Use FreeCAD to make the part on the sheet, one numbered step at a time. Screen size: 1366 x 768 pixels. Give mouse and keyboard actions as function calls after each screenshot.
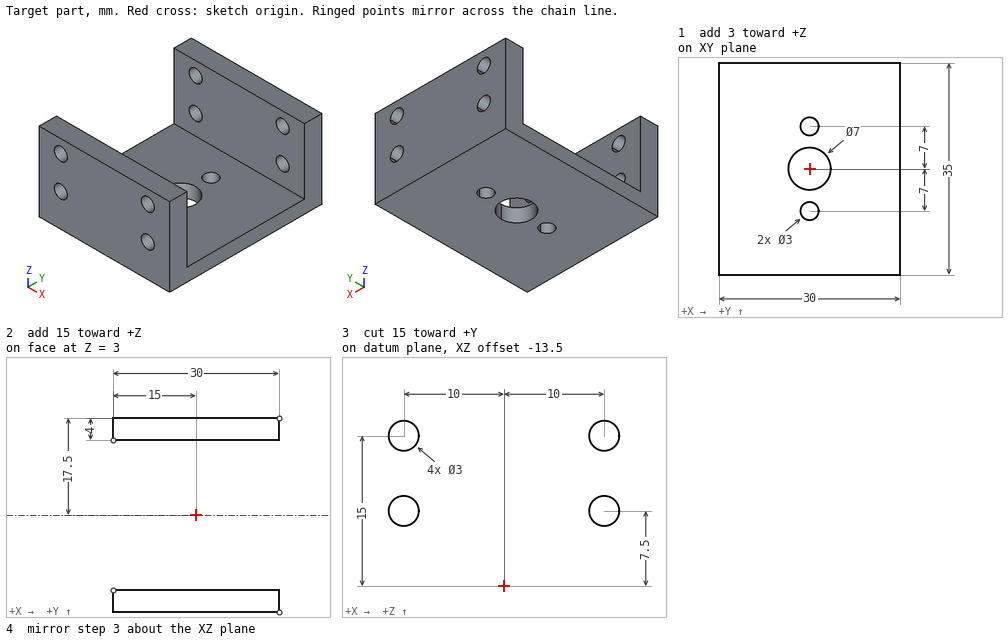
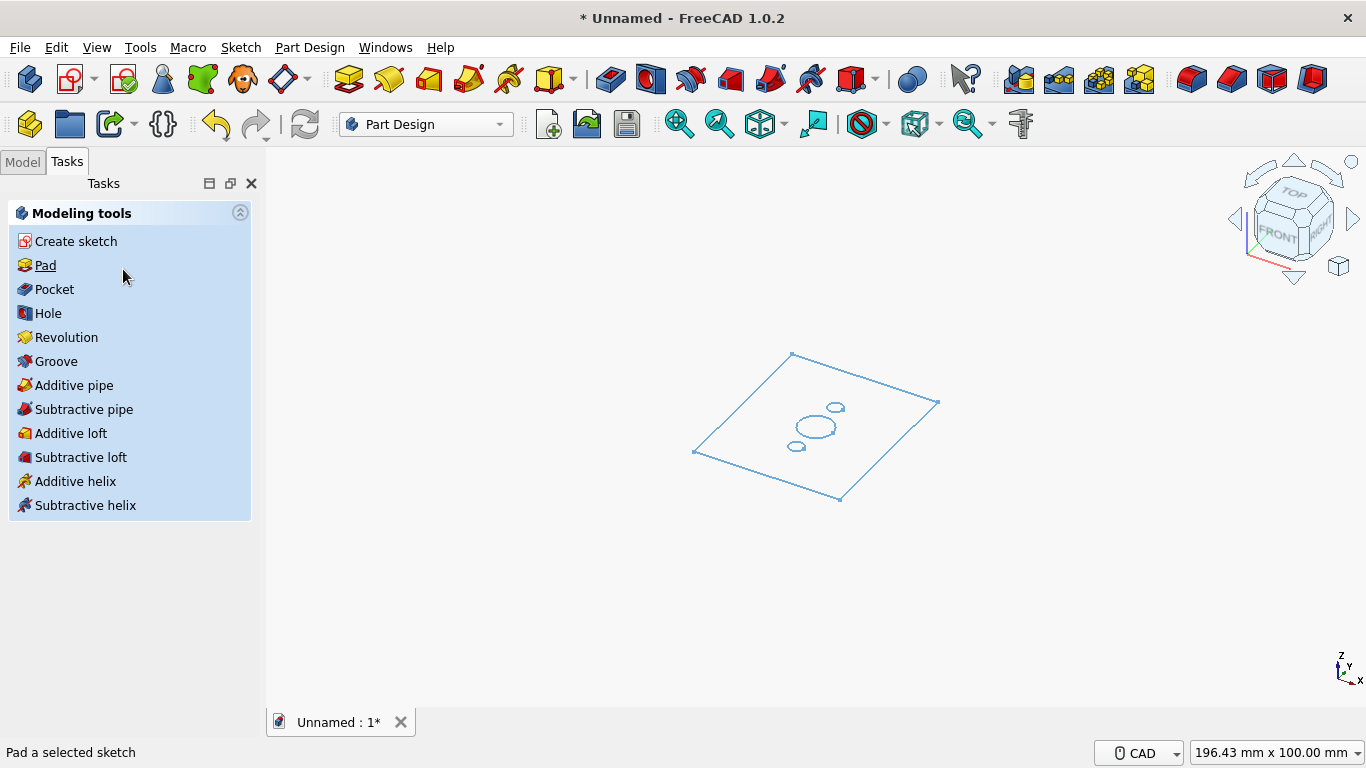
click(350, 80)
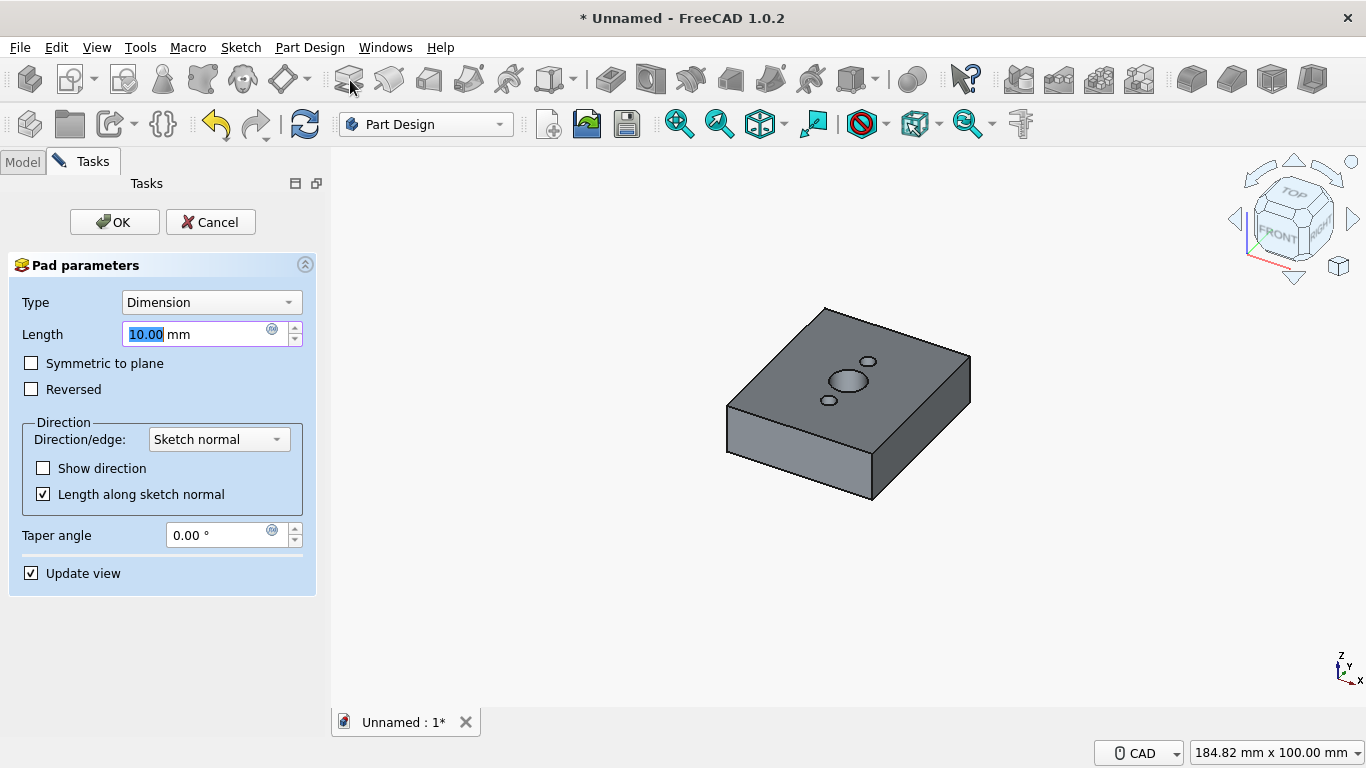
text(3)
key(Tab)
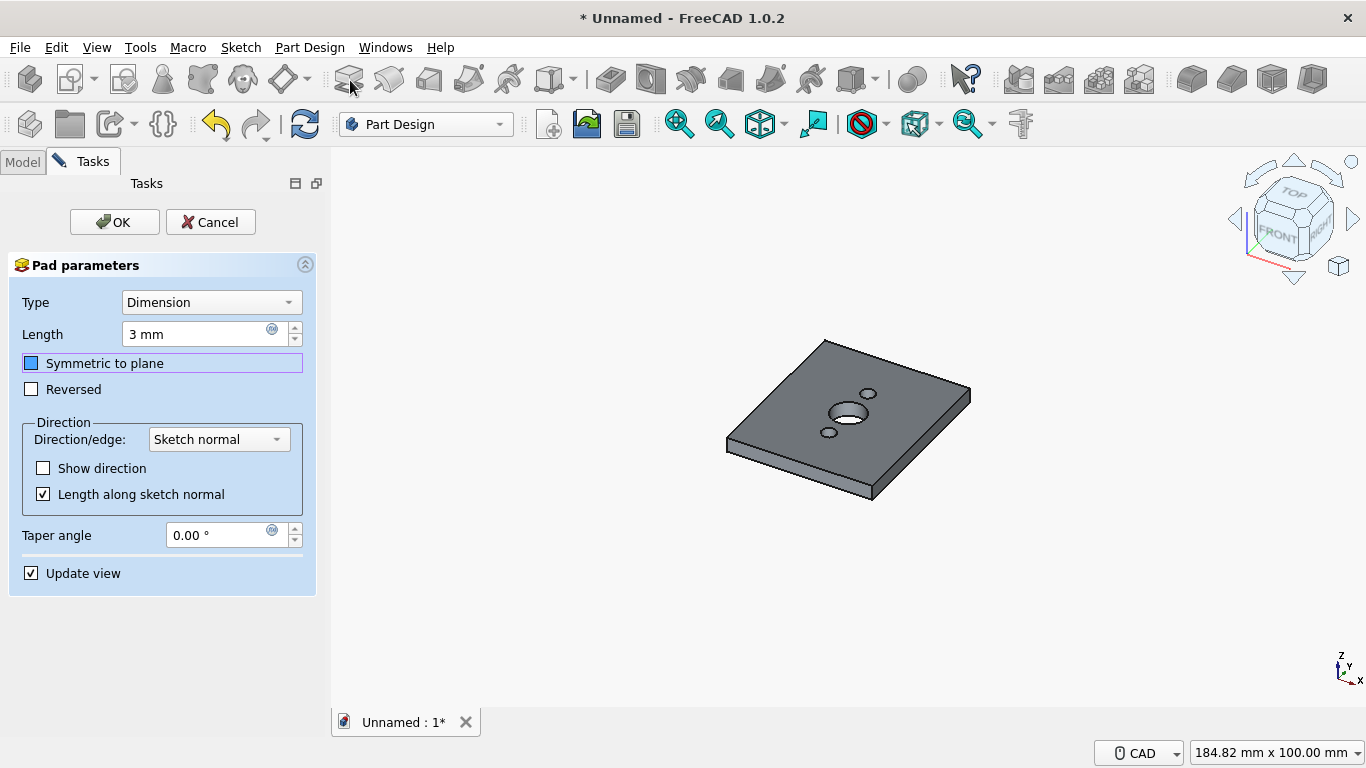
click(115, 222)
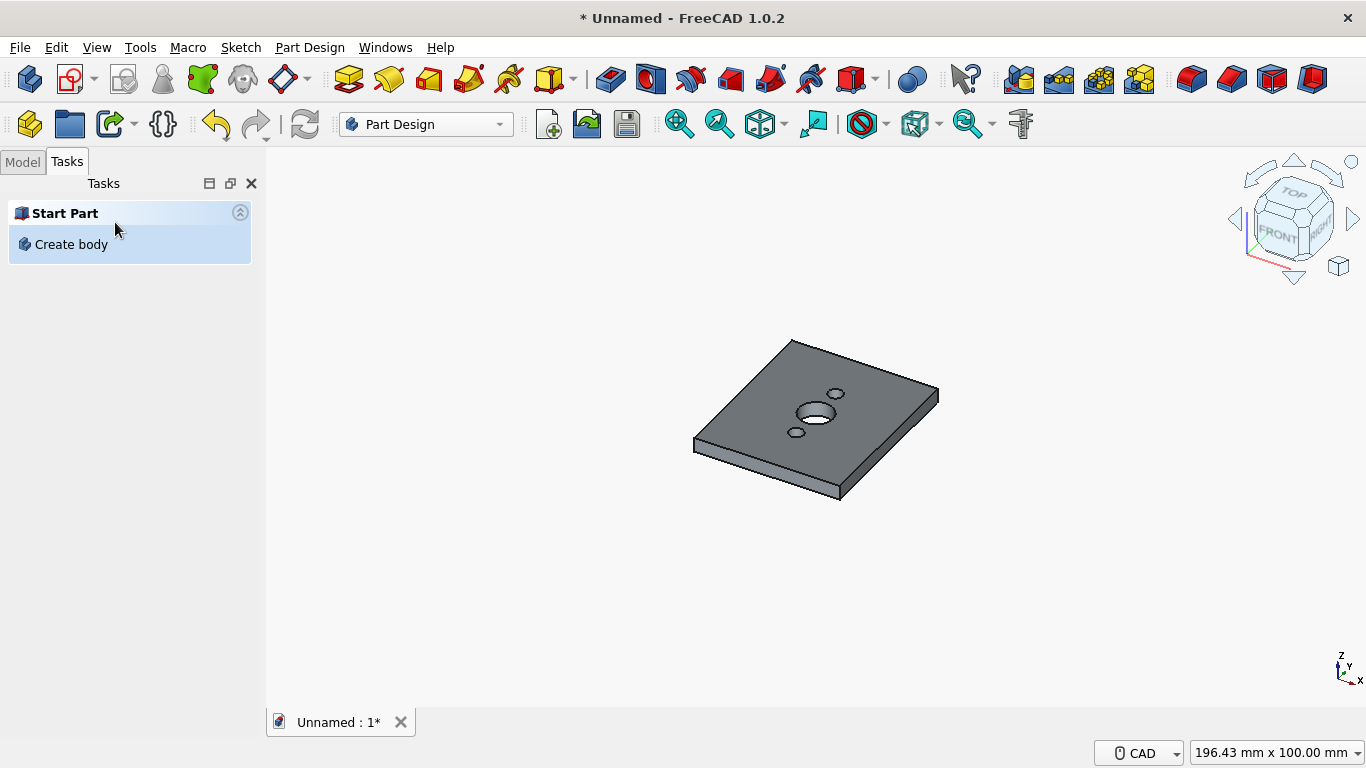
click(680, 124)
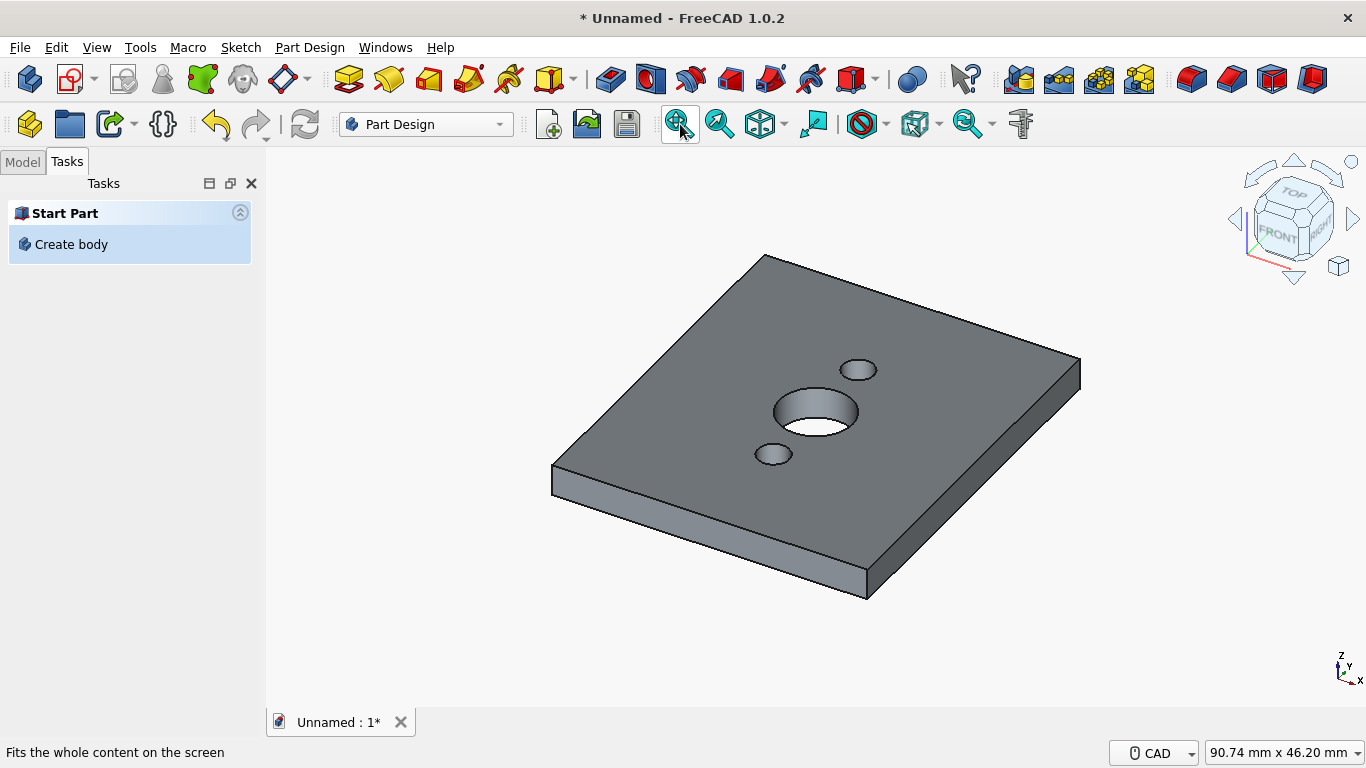
click(787, 321)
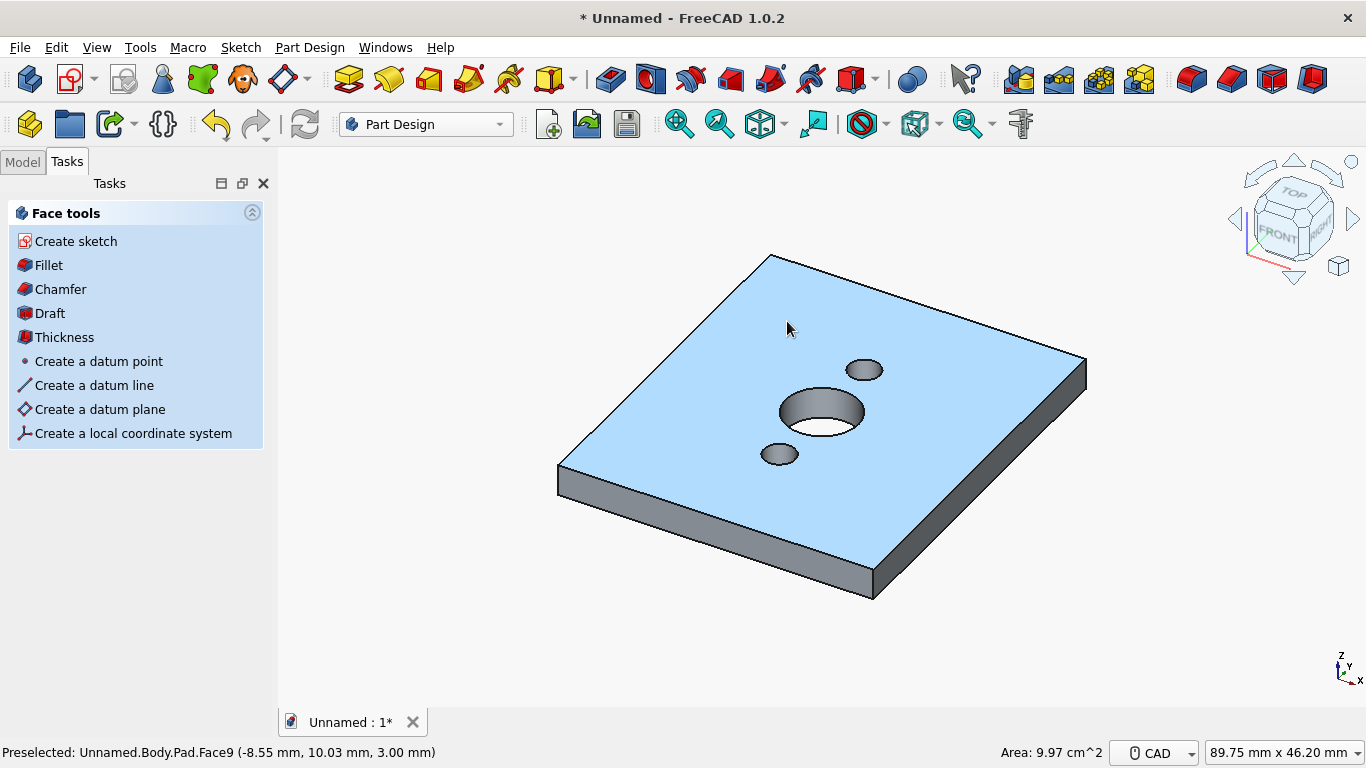
click(70, 80)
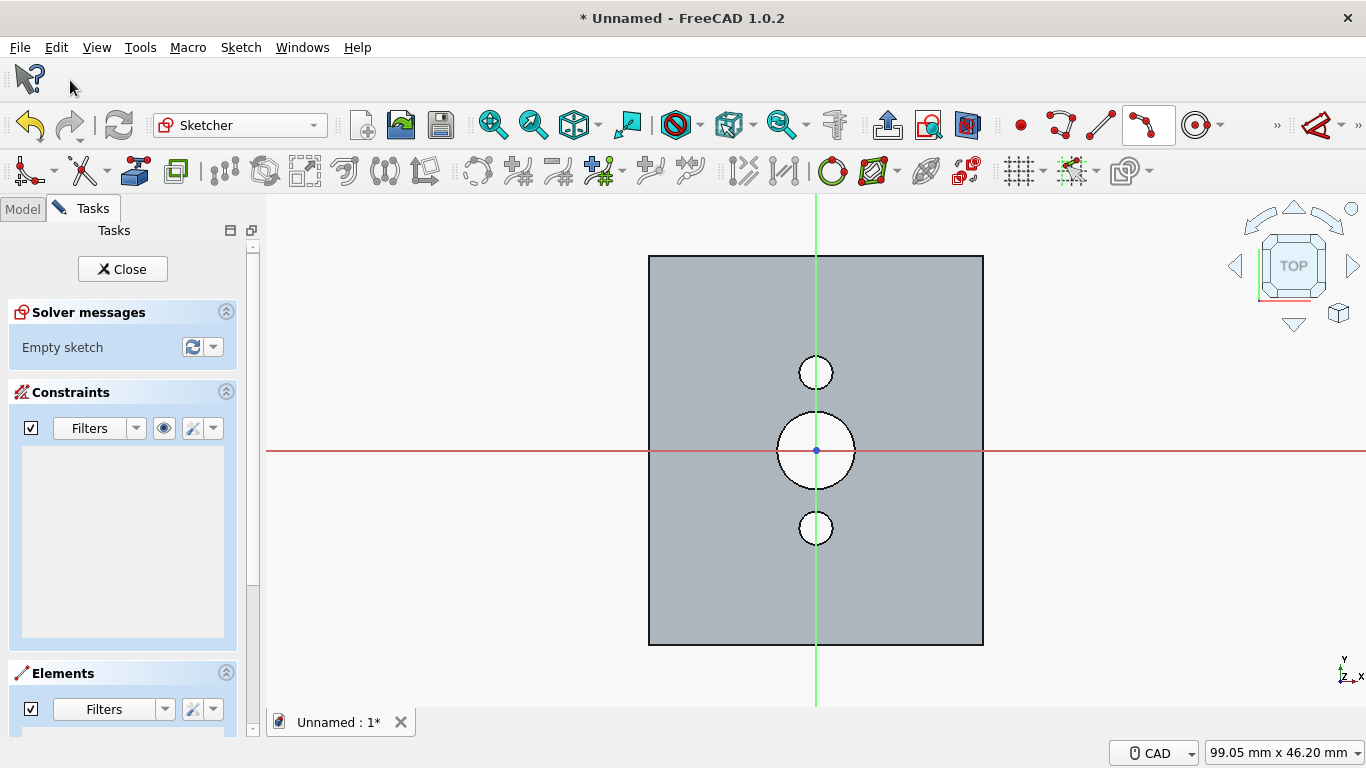
key(g)
key(r)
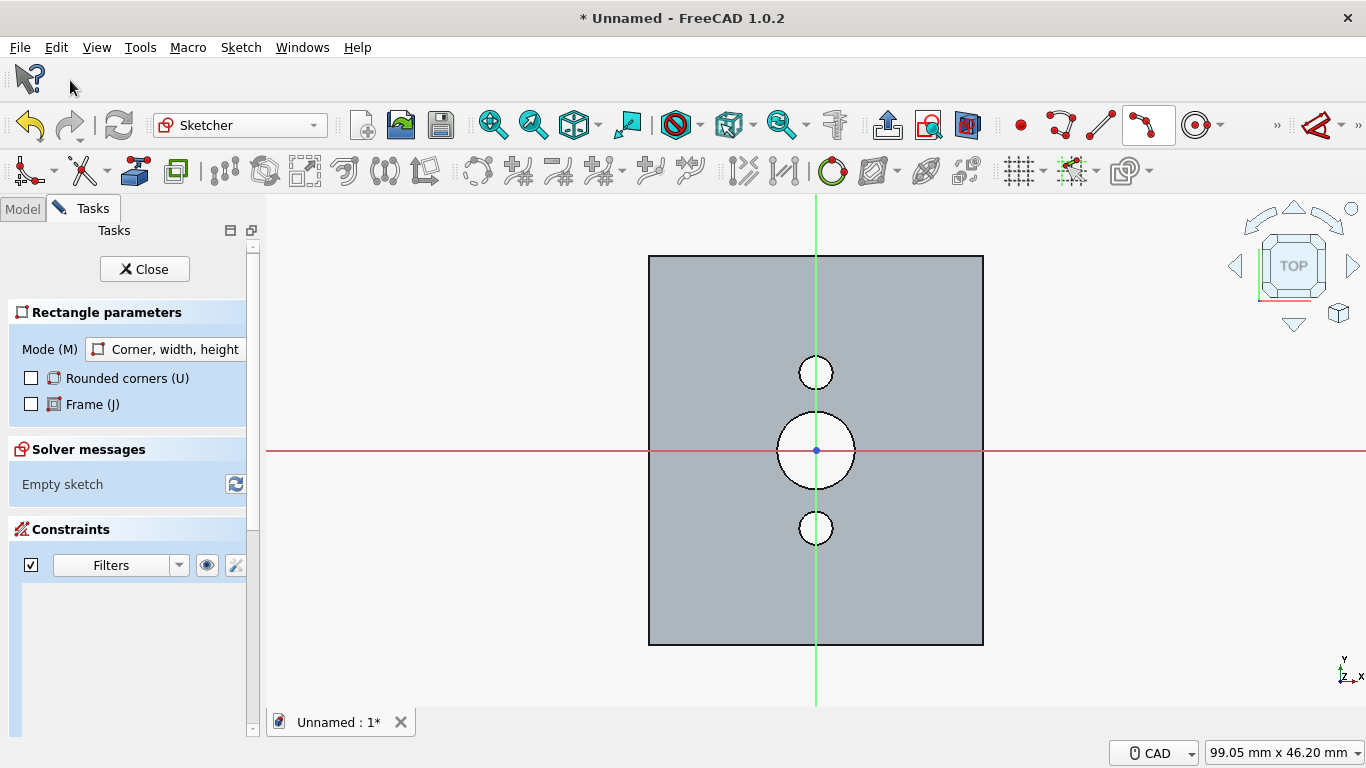
click(649, 256)
click(983, 301)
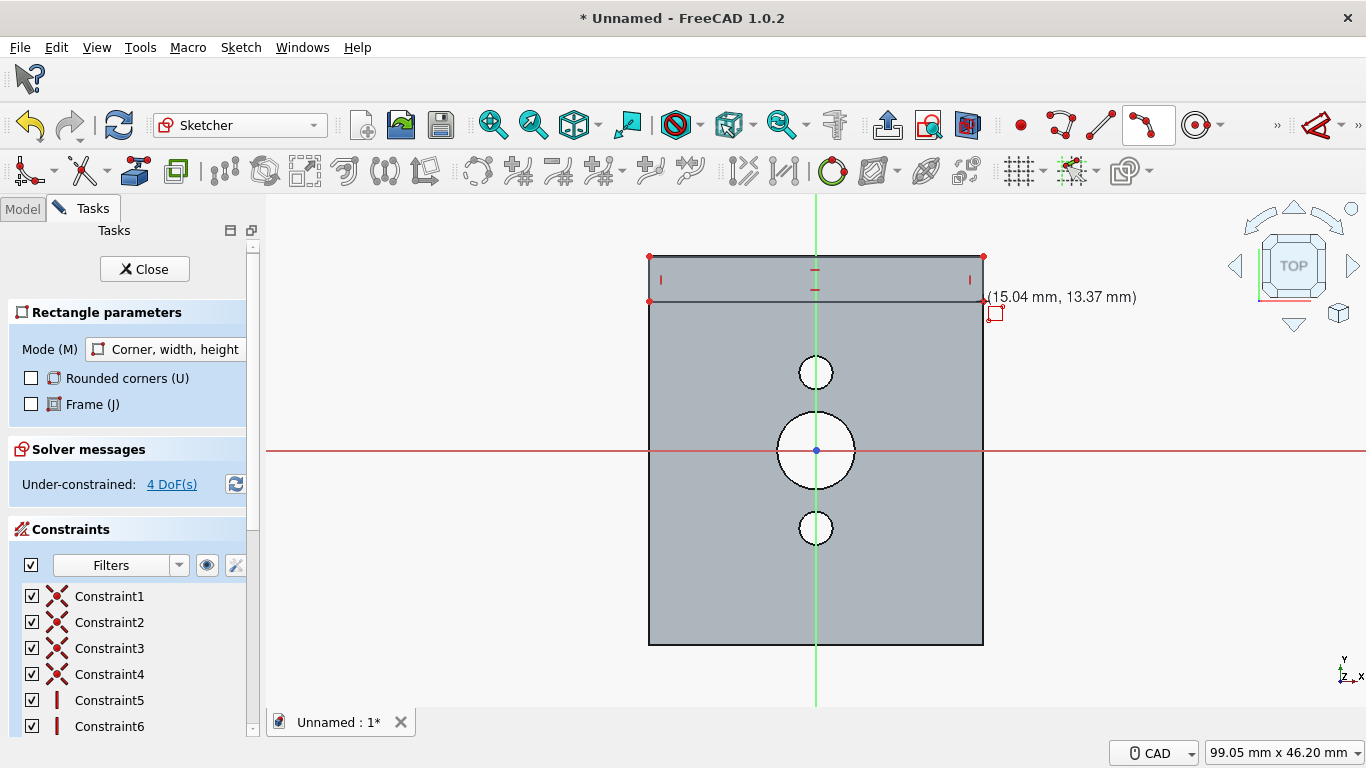
click(649, 600)
click(983, 645)
key(Escape)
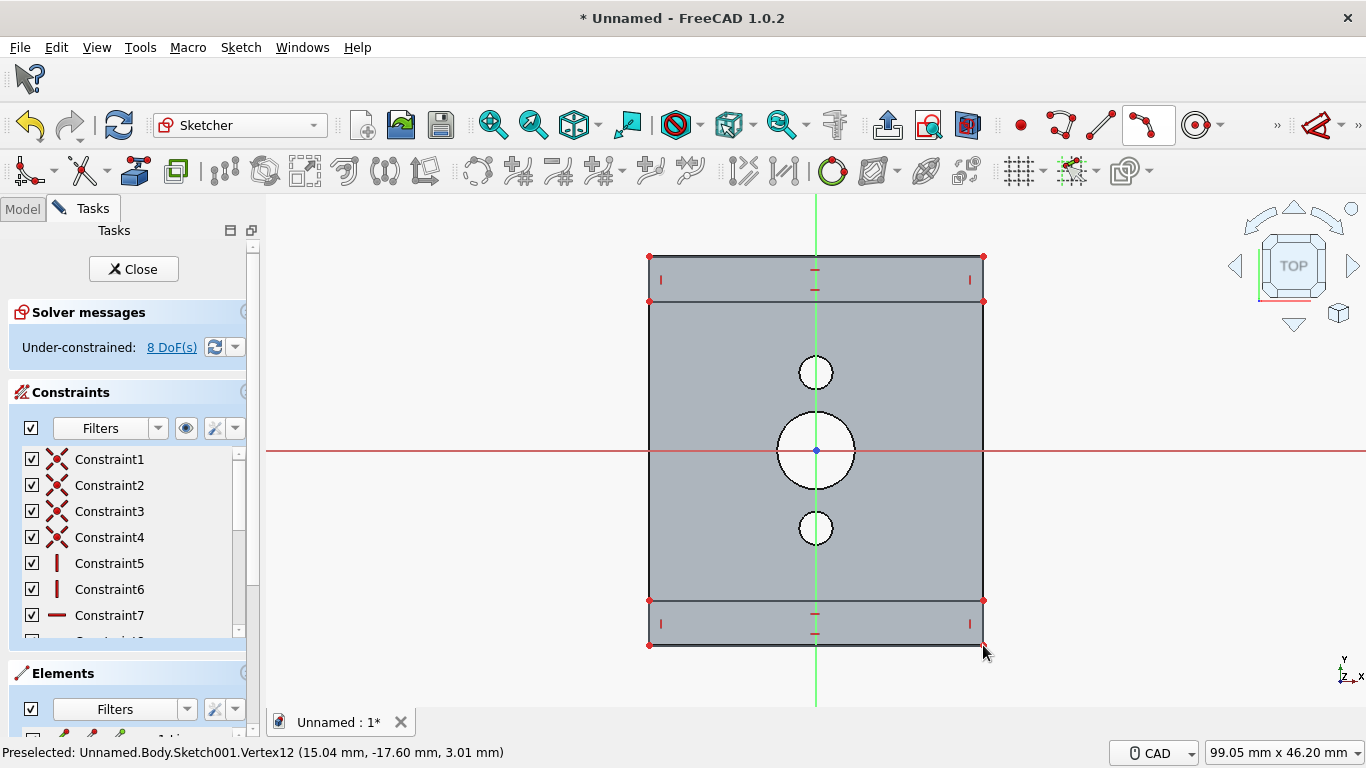
click(649, 302)